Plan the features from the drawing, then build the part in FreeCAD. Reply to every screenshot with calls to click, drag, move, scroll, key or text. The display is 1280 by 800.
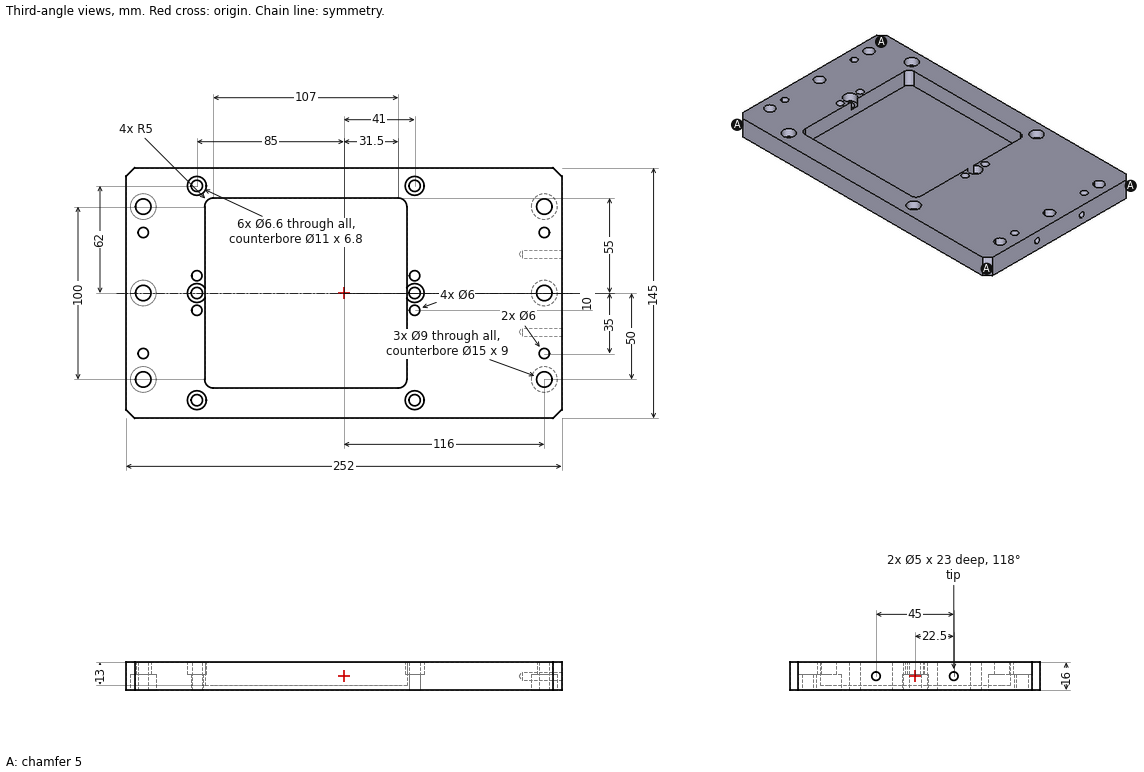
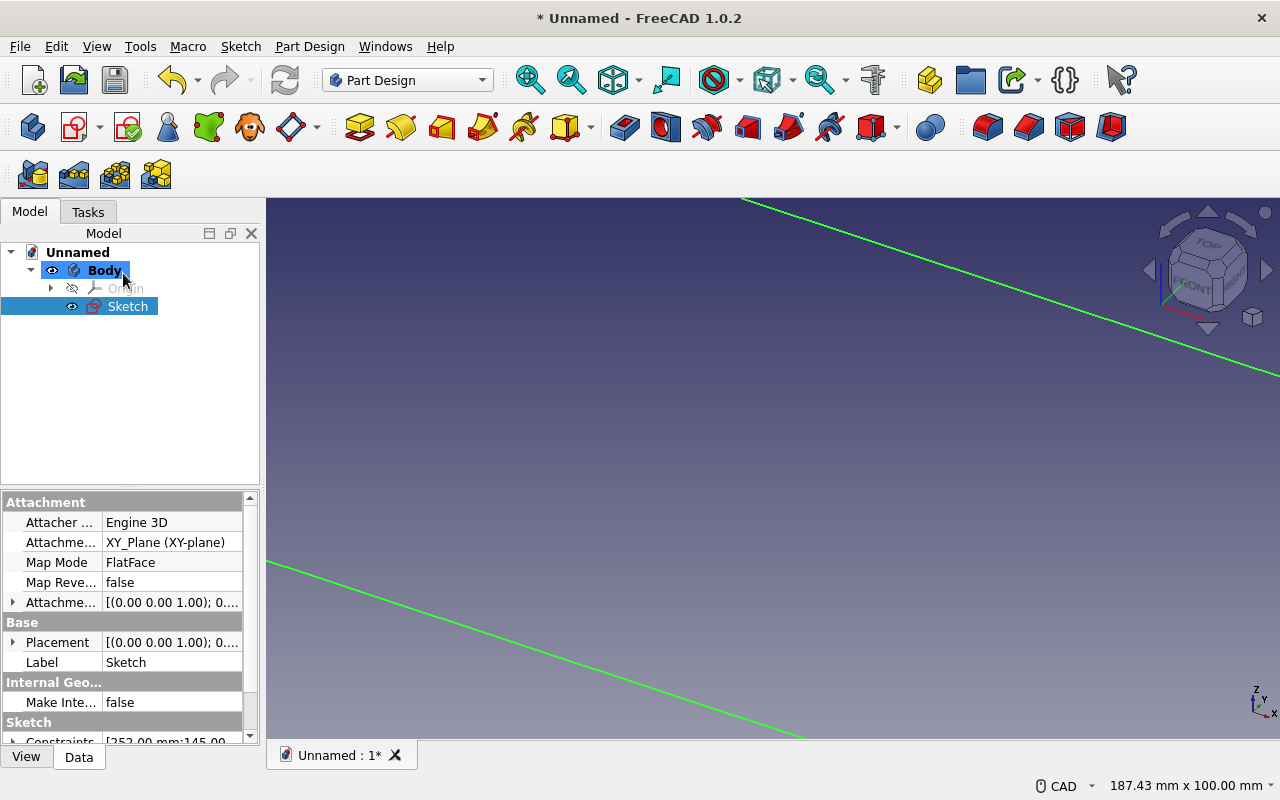
click(360, 128)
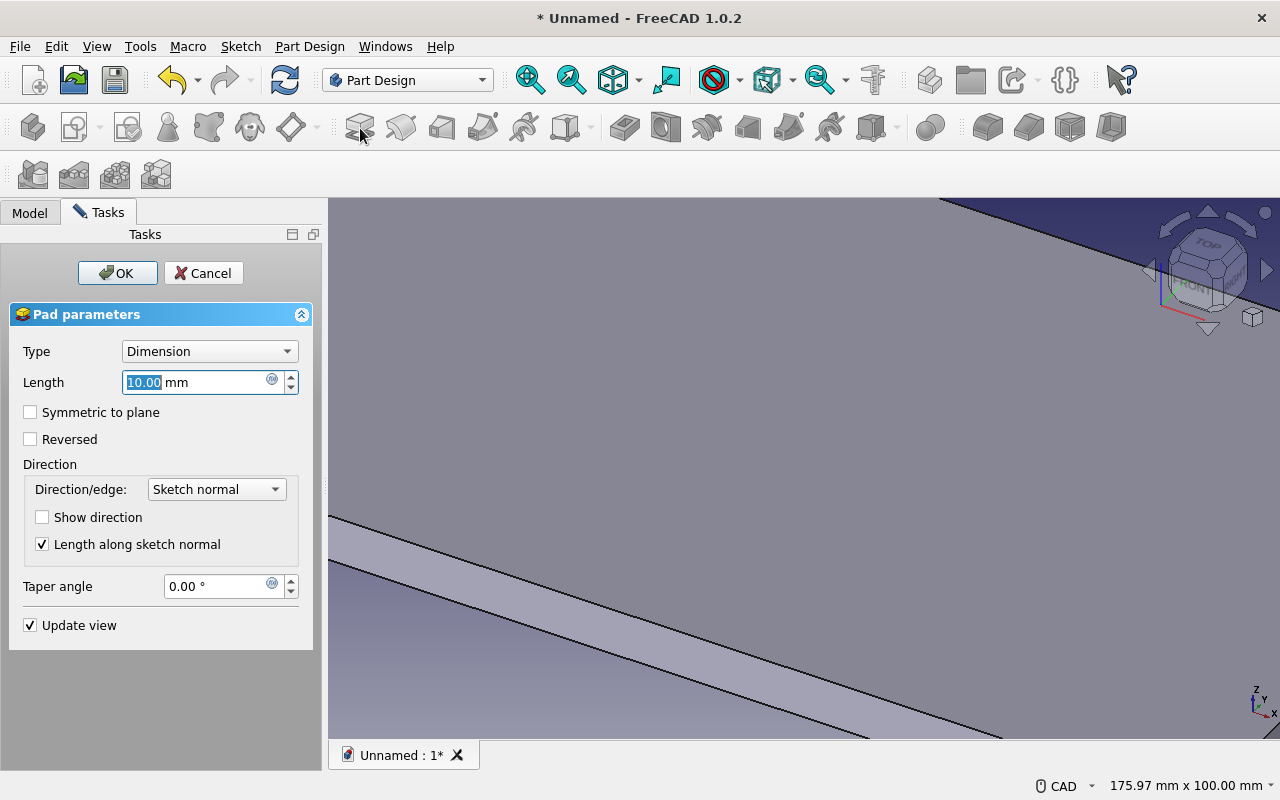
text(16)
key(Tab)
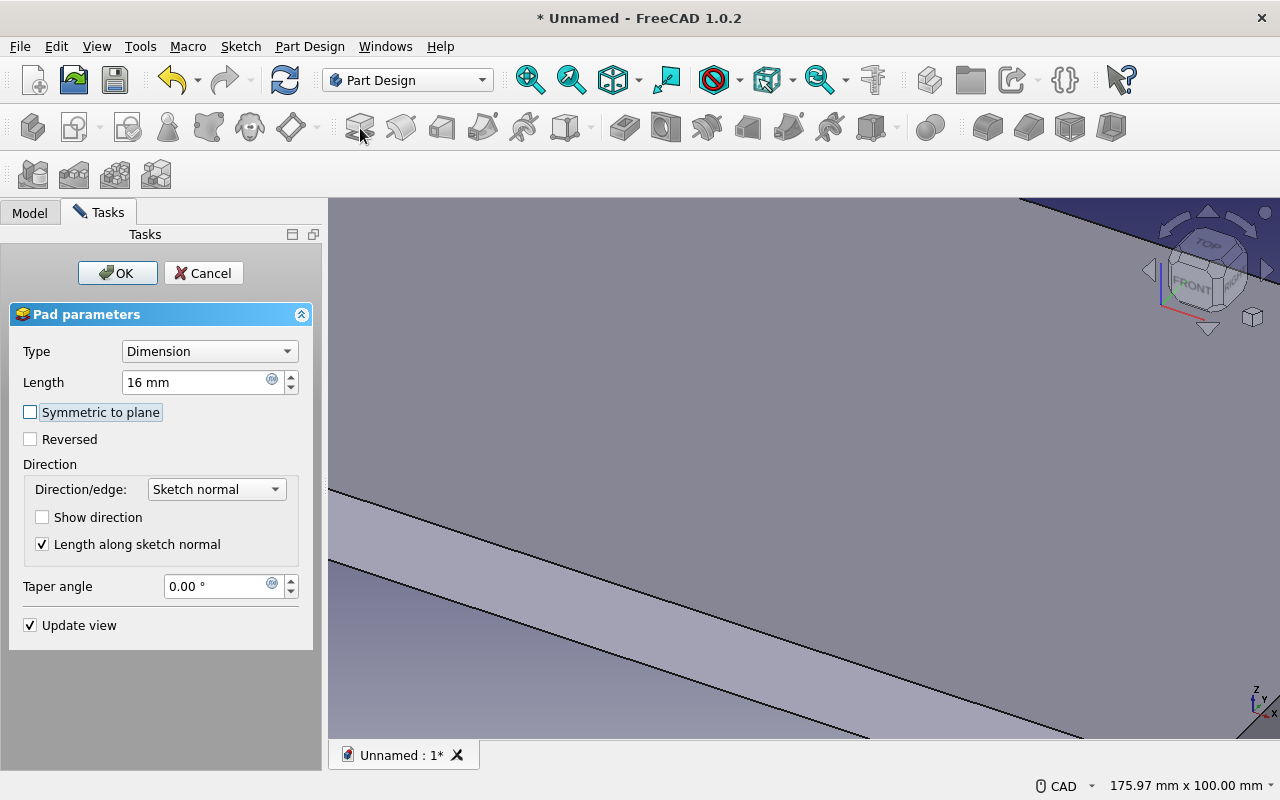
click(31, 412)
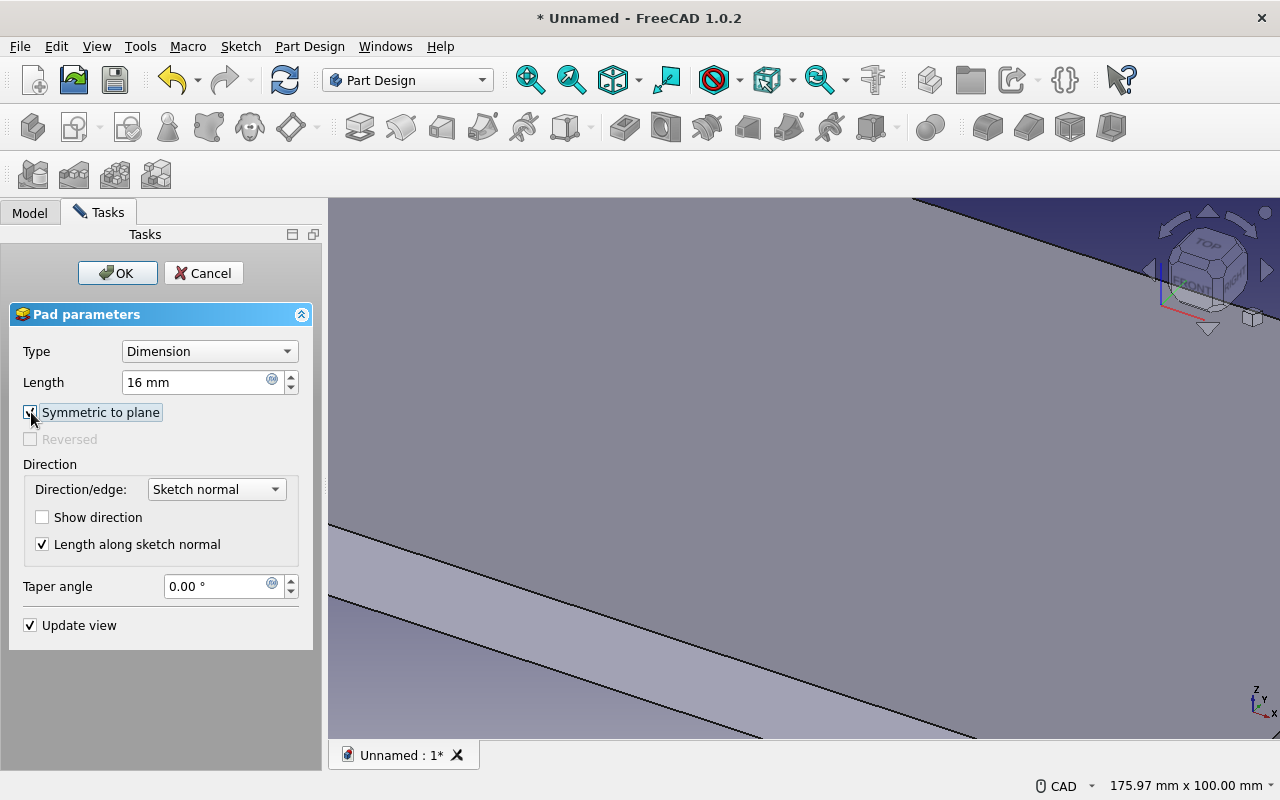
click(118, 273)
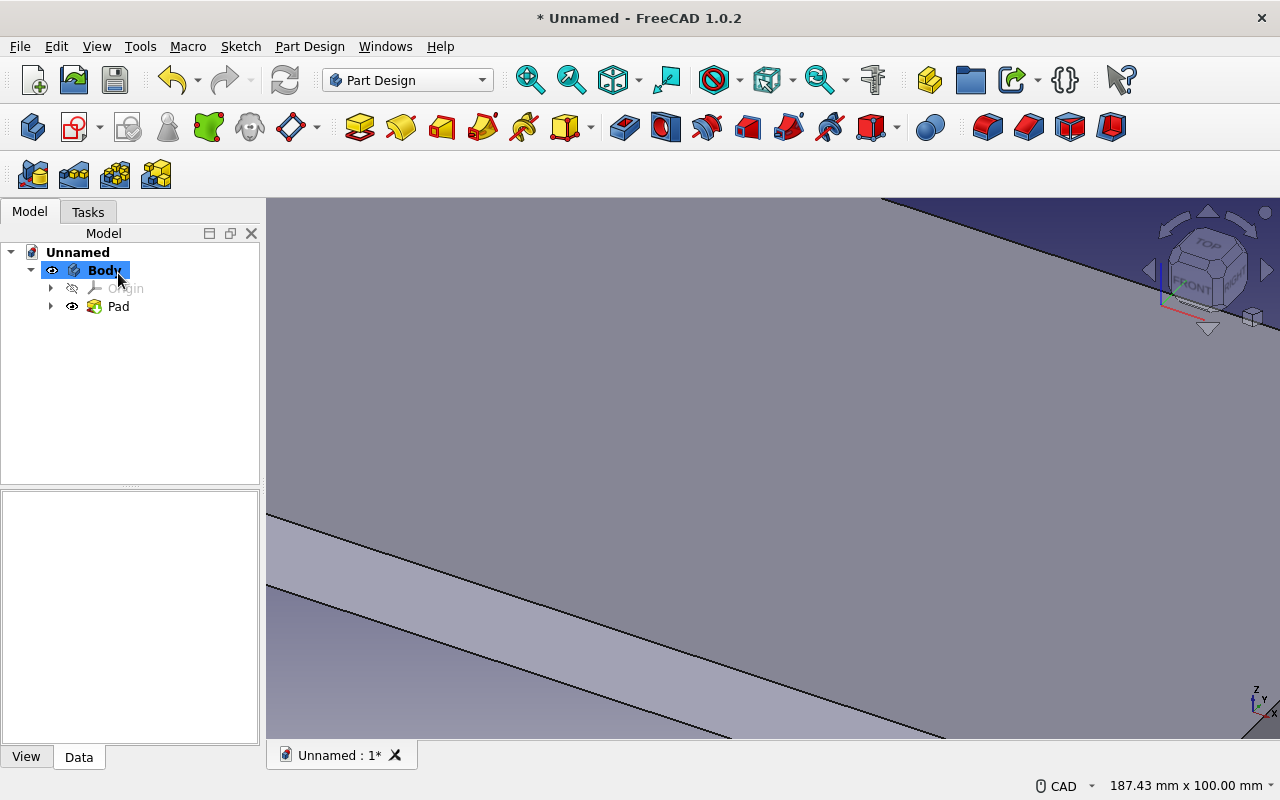
click(531, 80)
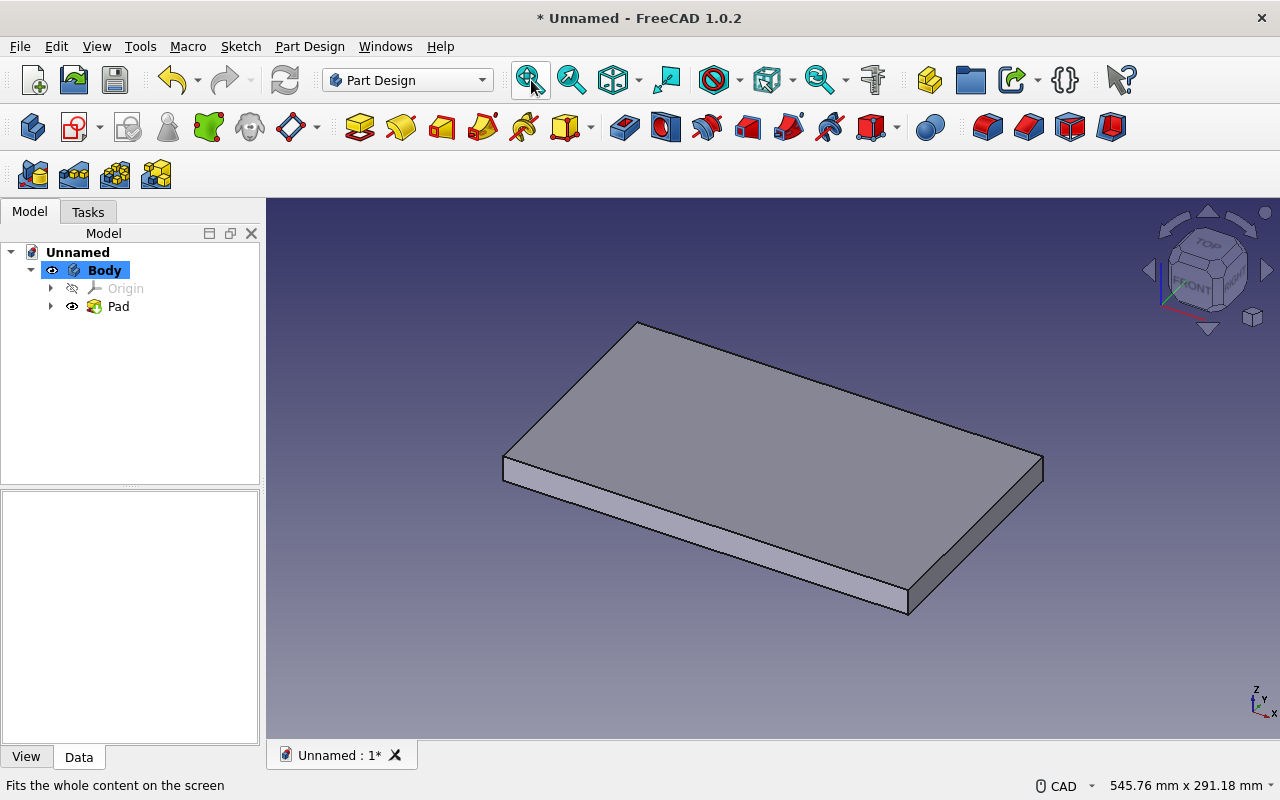
click(831, 475)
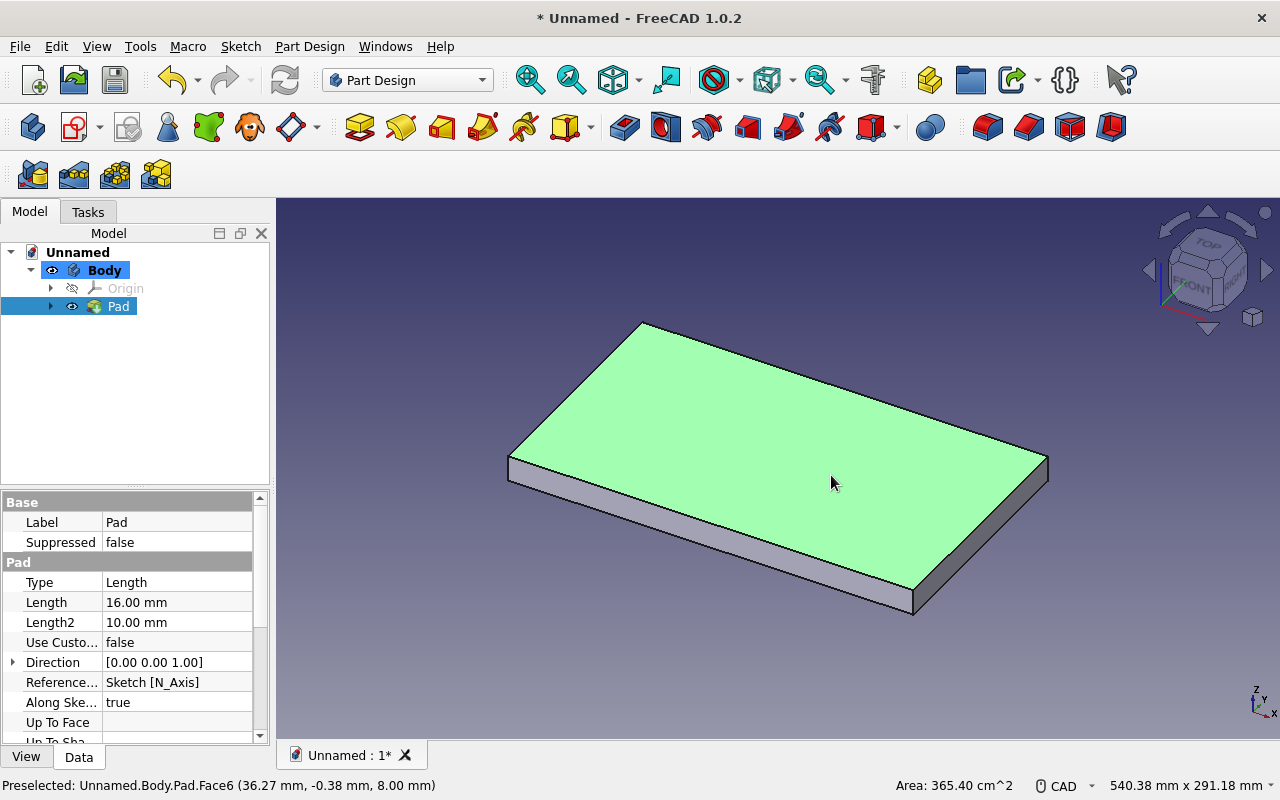
click(74, 128)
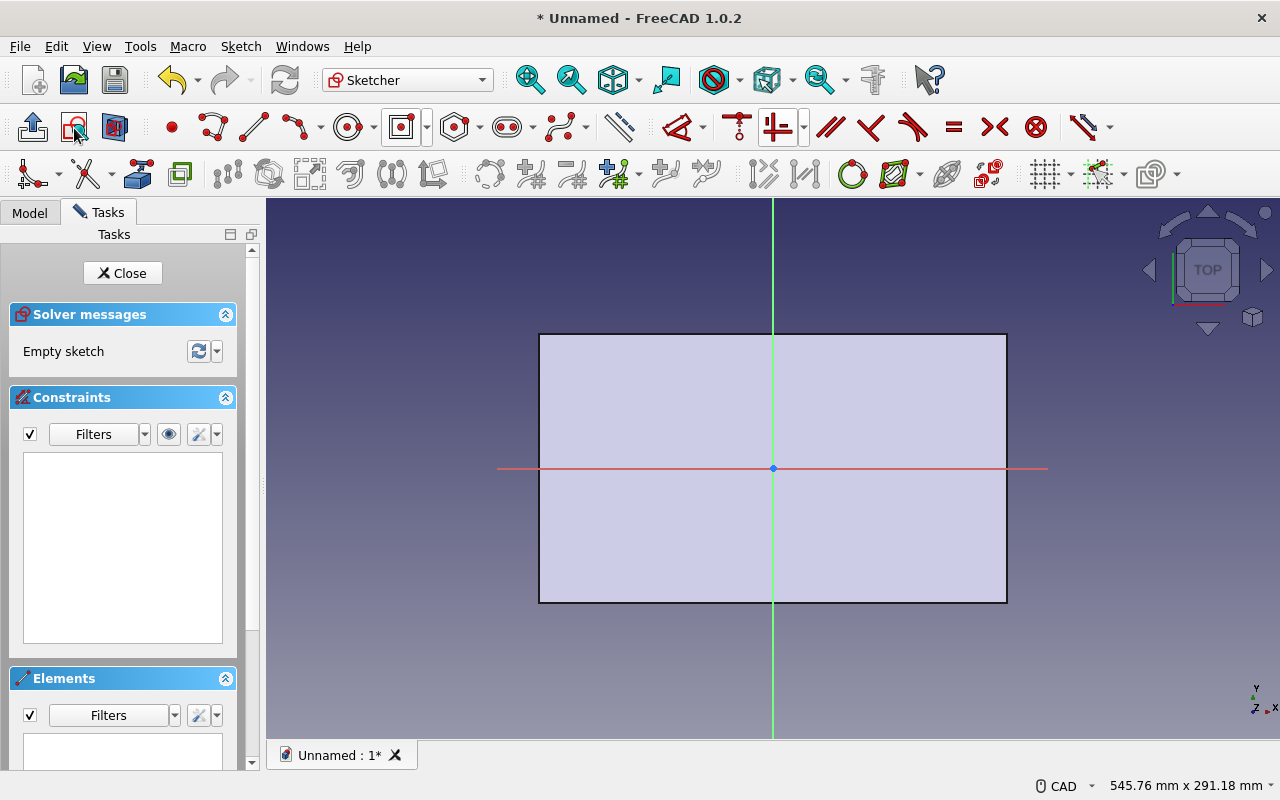
scroll(788, 469, up, 2)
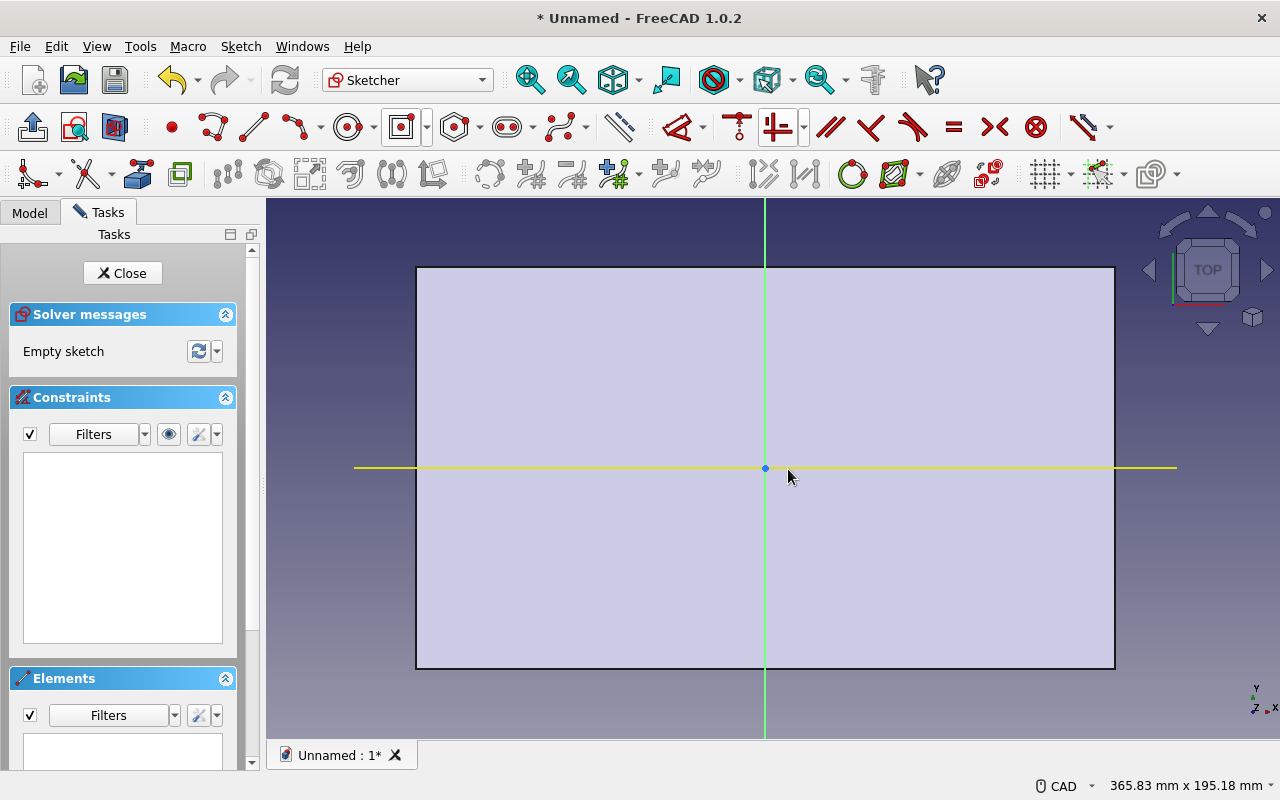
key(g)
key(c)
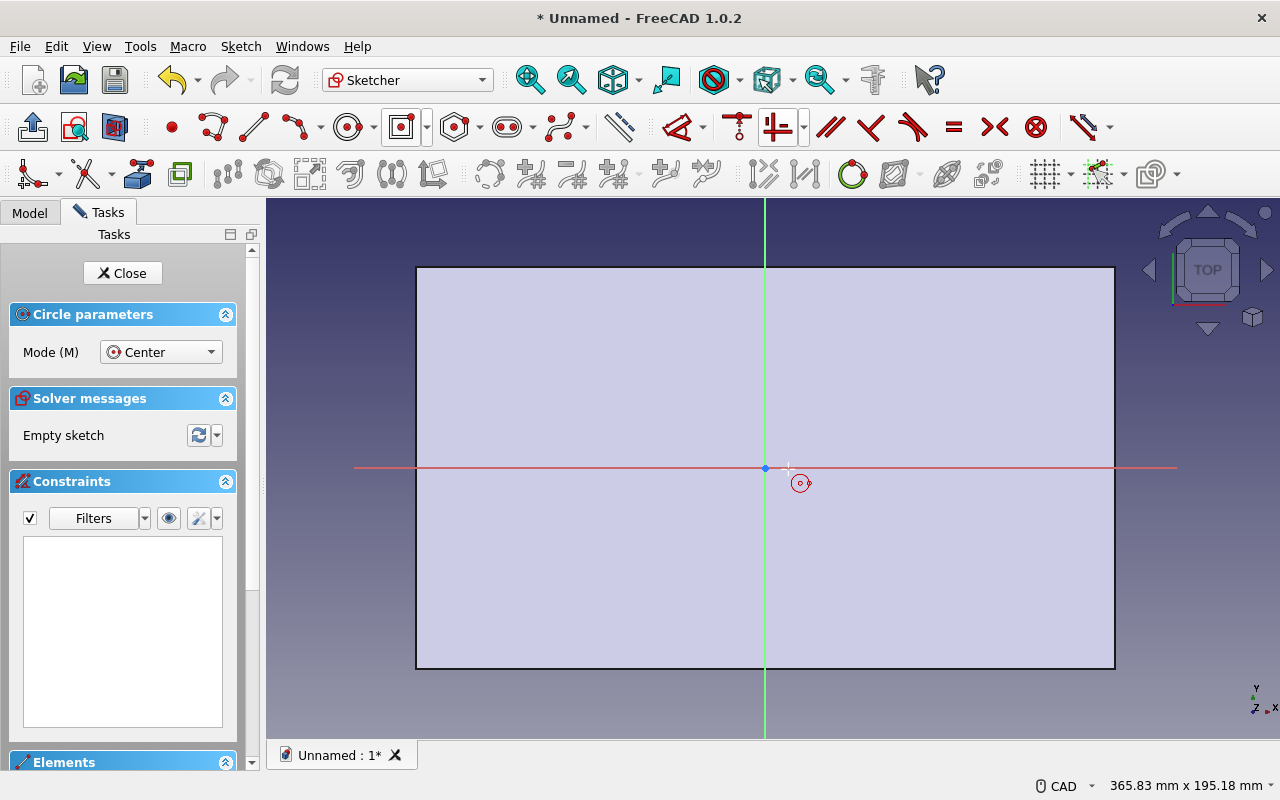
scroll(530, 296, up, 5)